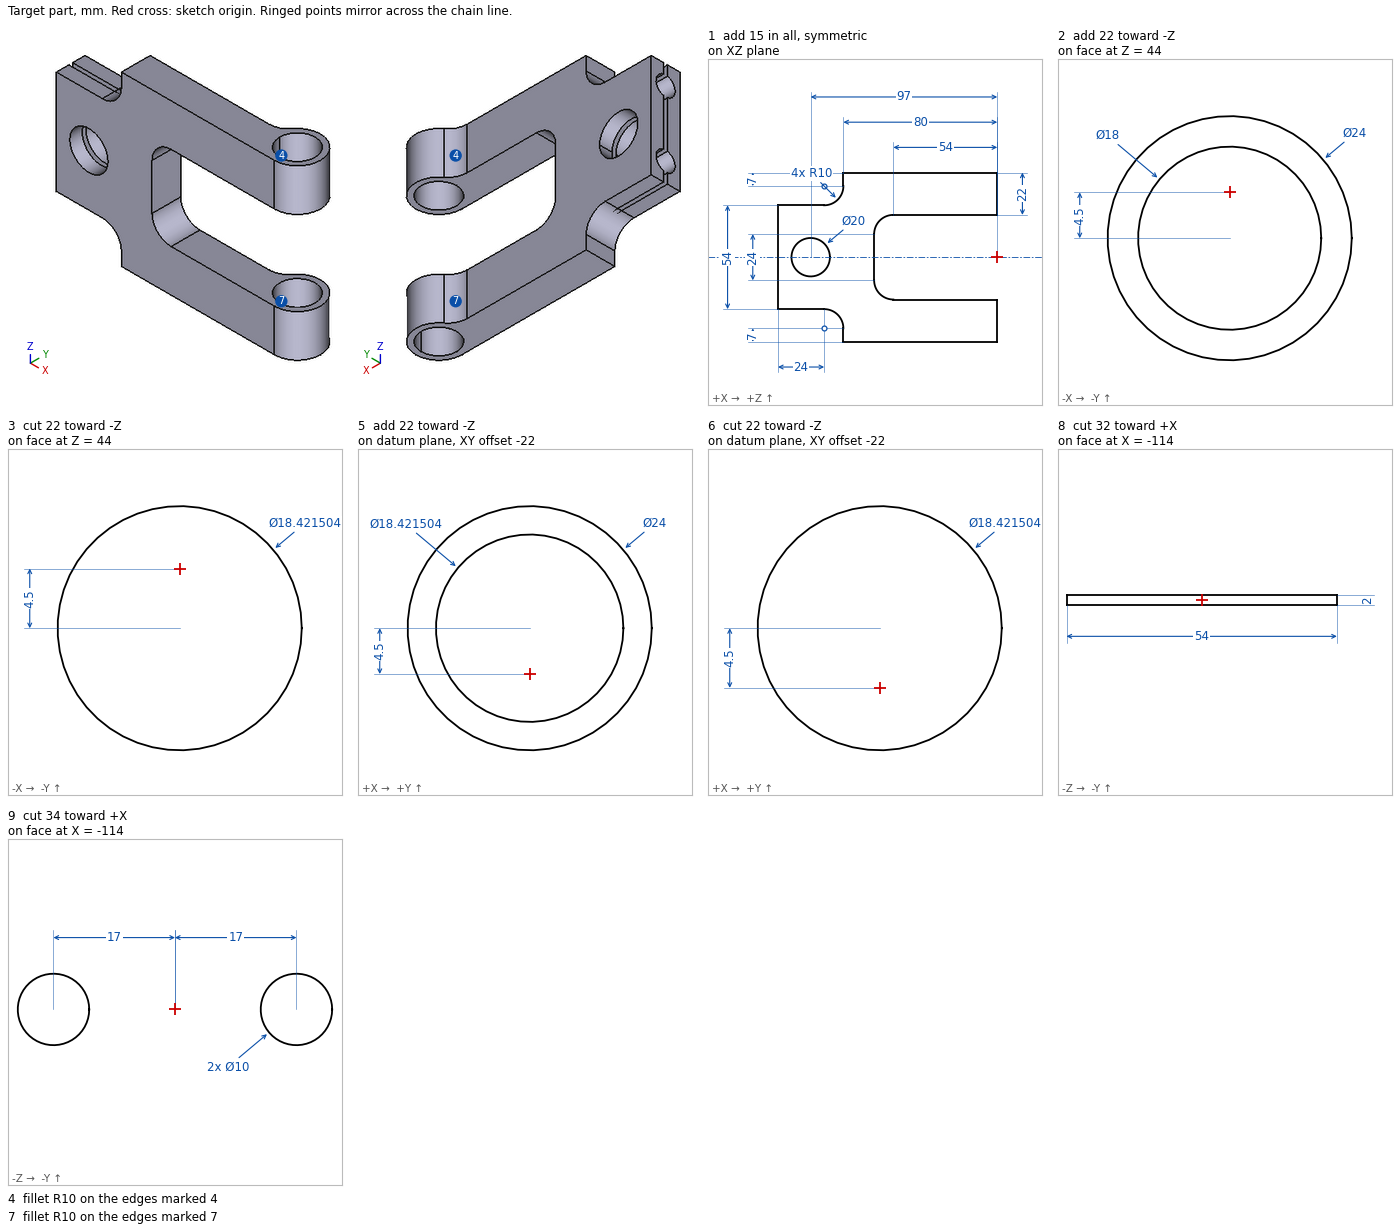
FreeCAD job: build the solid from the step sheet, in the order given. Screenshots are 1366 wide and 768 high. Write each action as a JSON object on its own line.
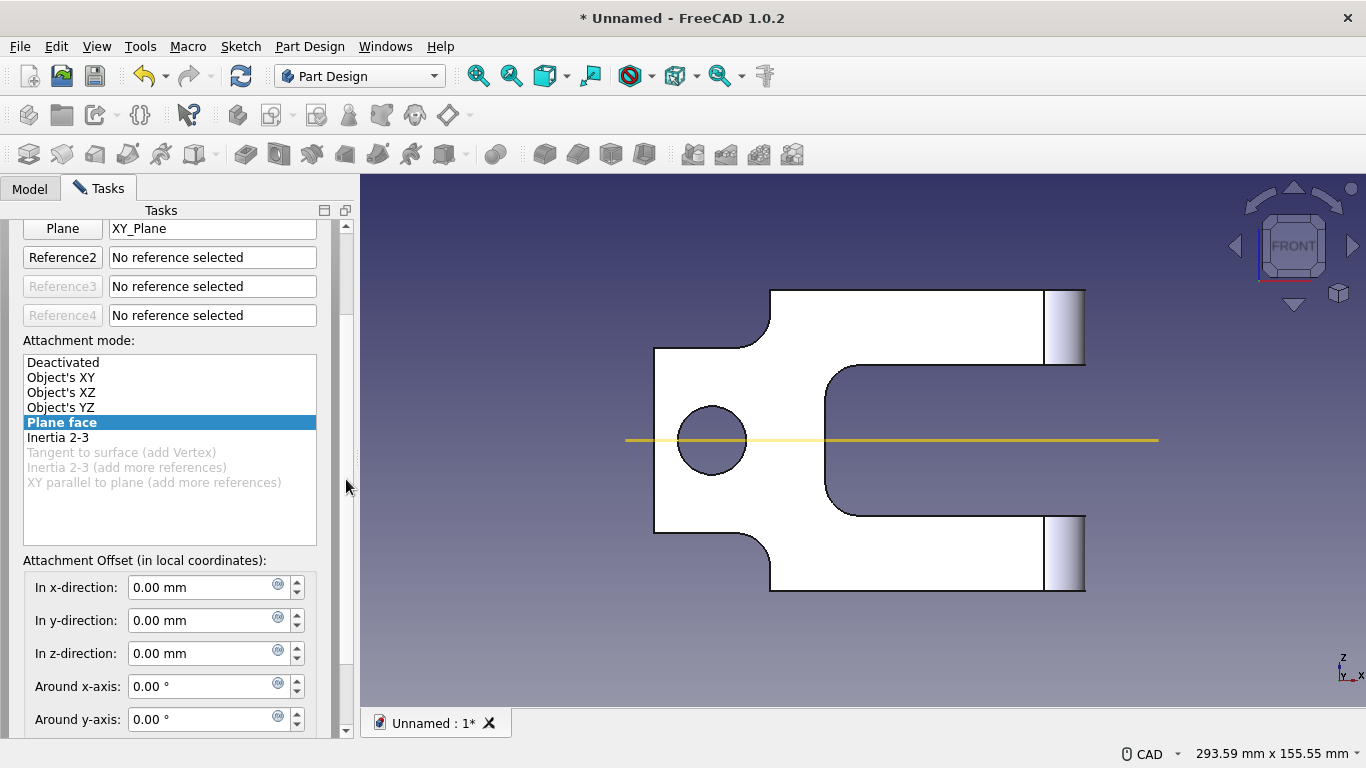
{"action": "triple_click", "coordinate": [210, 654]}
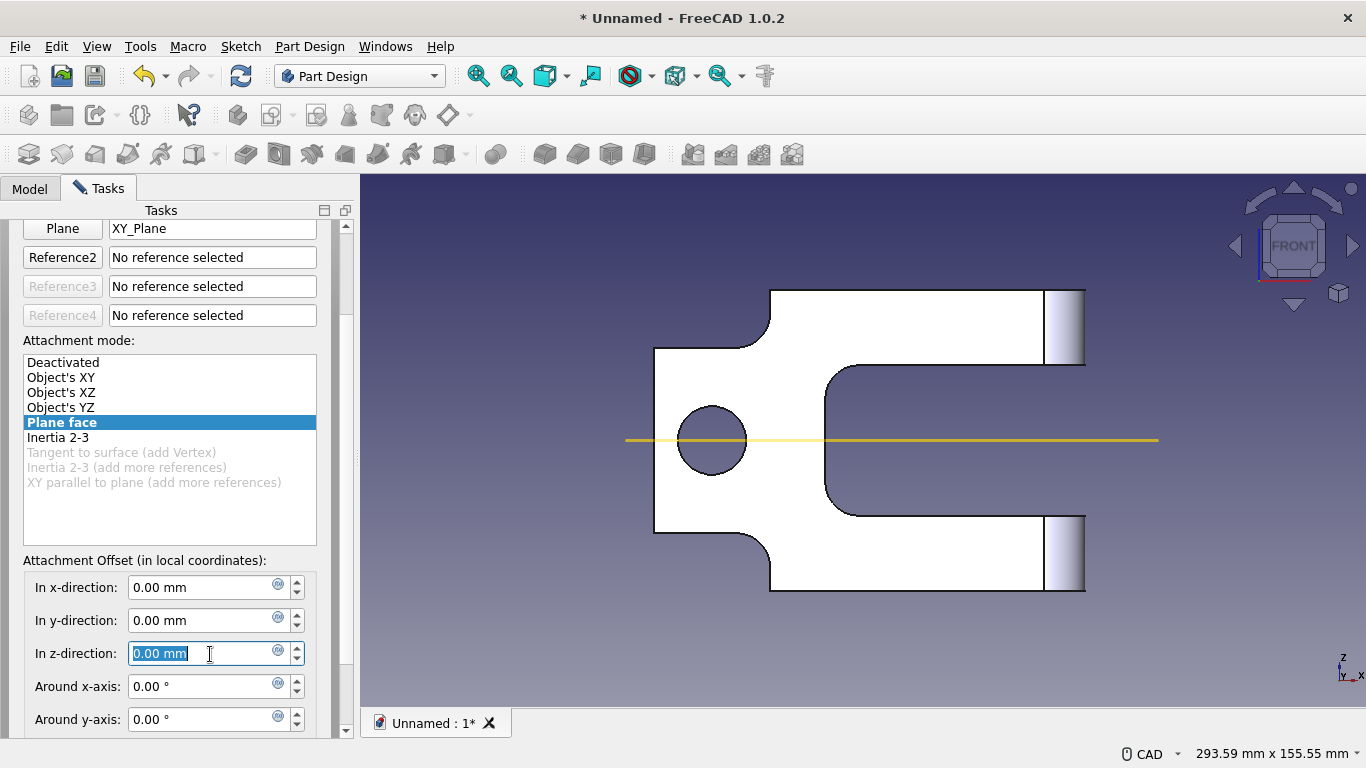
{"action": "type", "text": "-22"}
{"action": "key", "text": "Tab"}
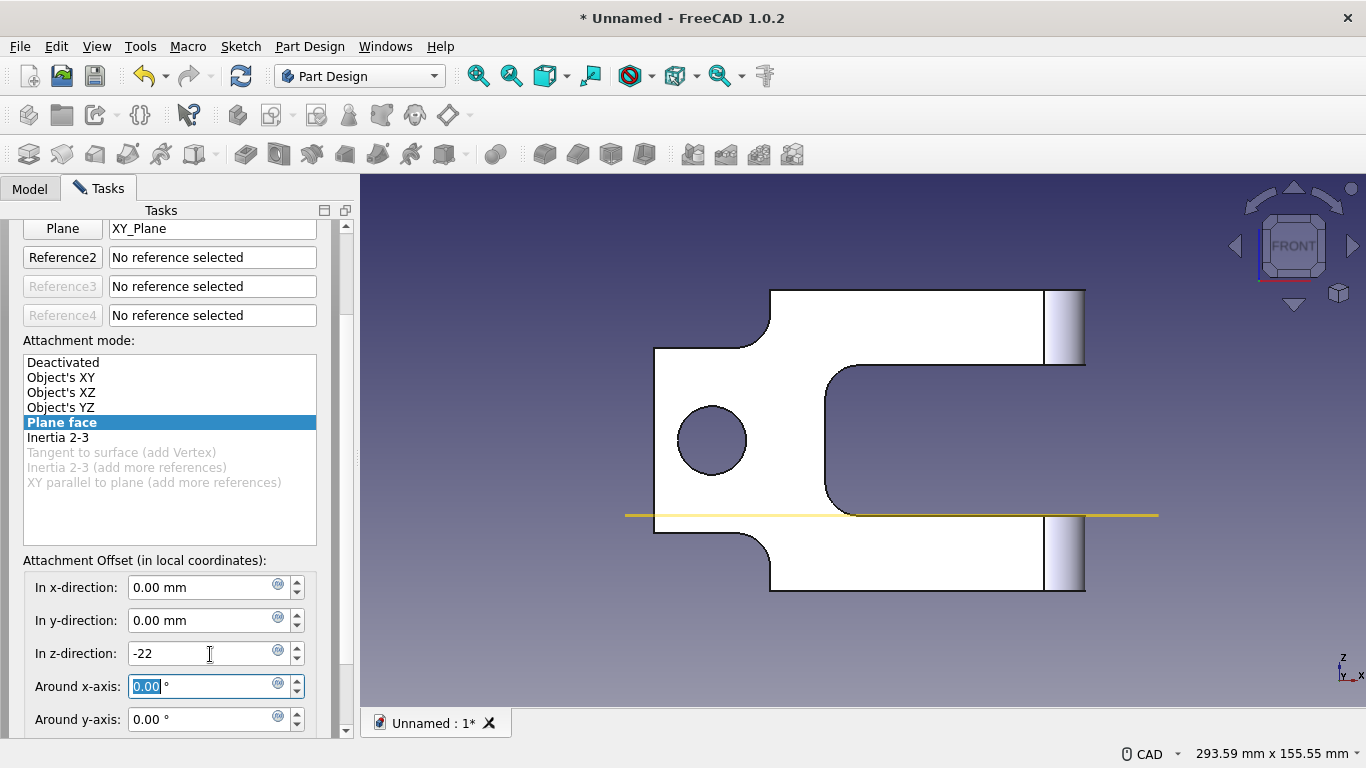
{"action": "scroll", "coordinate": [346, 479], "scroll_direction": "up", "scroll_amount": 3}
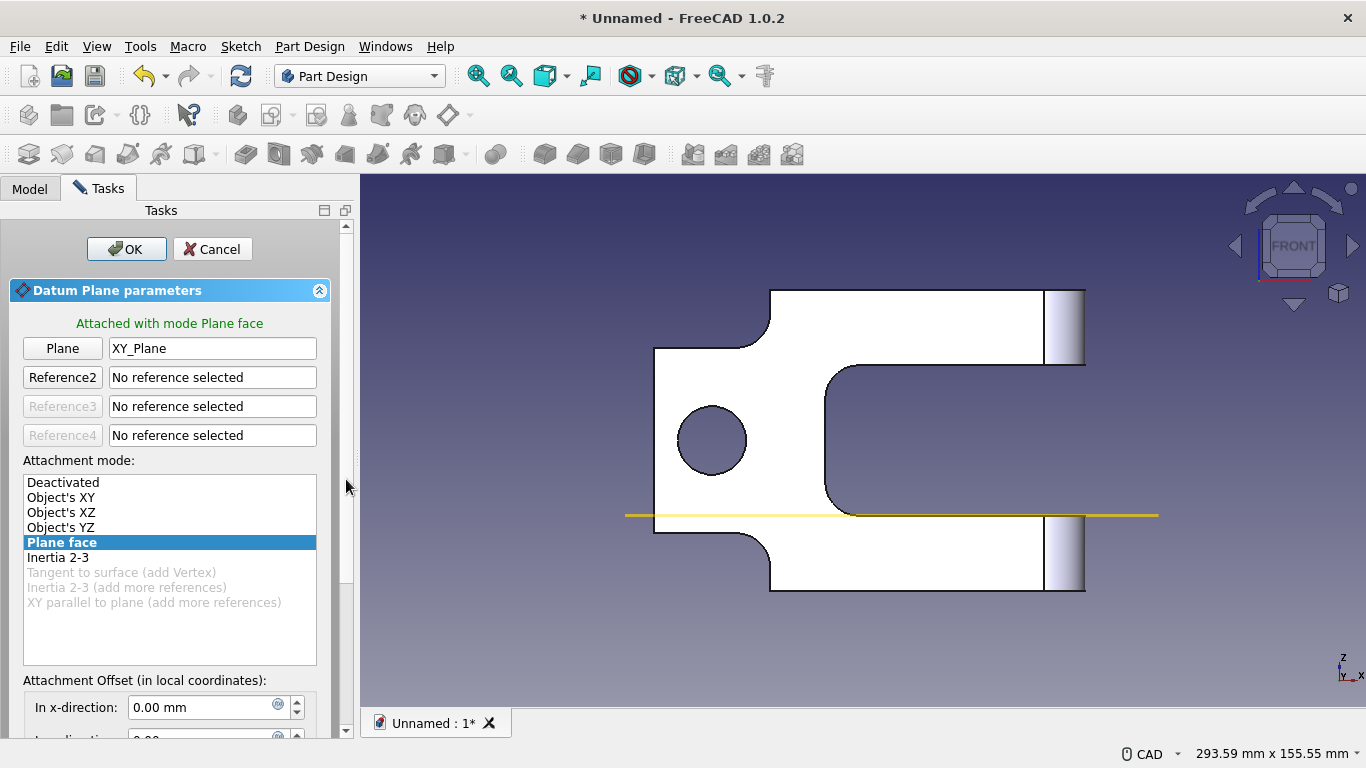
{"action": "left_click", "coordinate": [127, 249]}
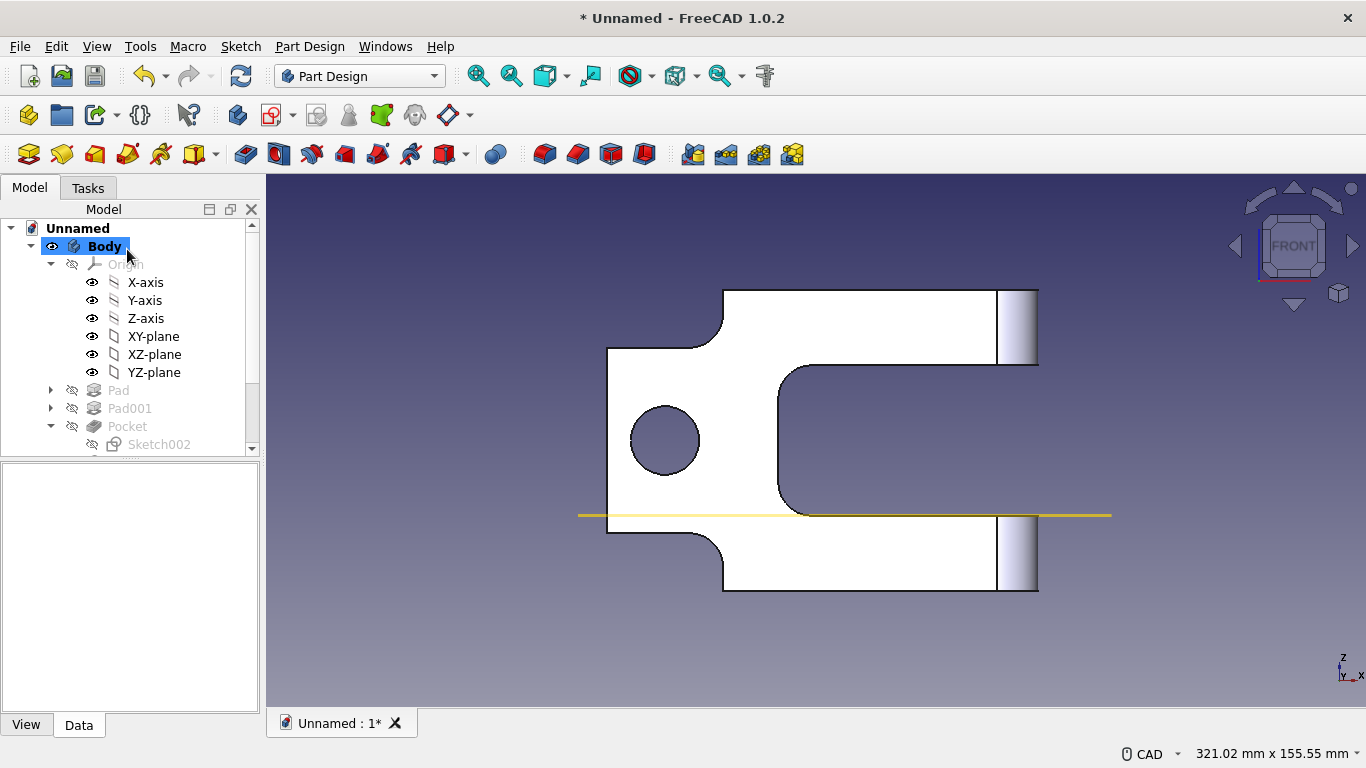
{"action": "scroll", "coordinate": [101, 332], "scroll_direction": "down", "scroll_amount": 3}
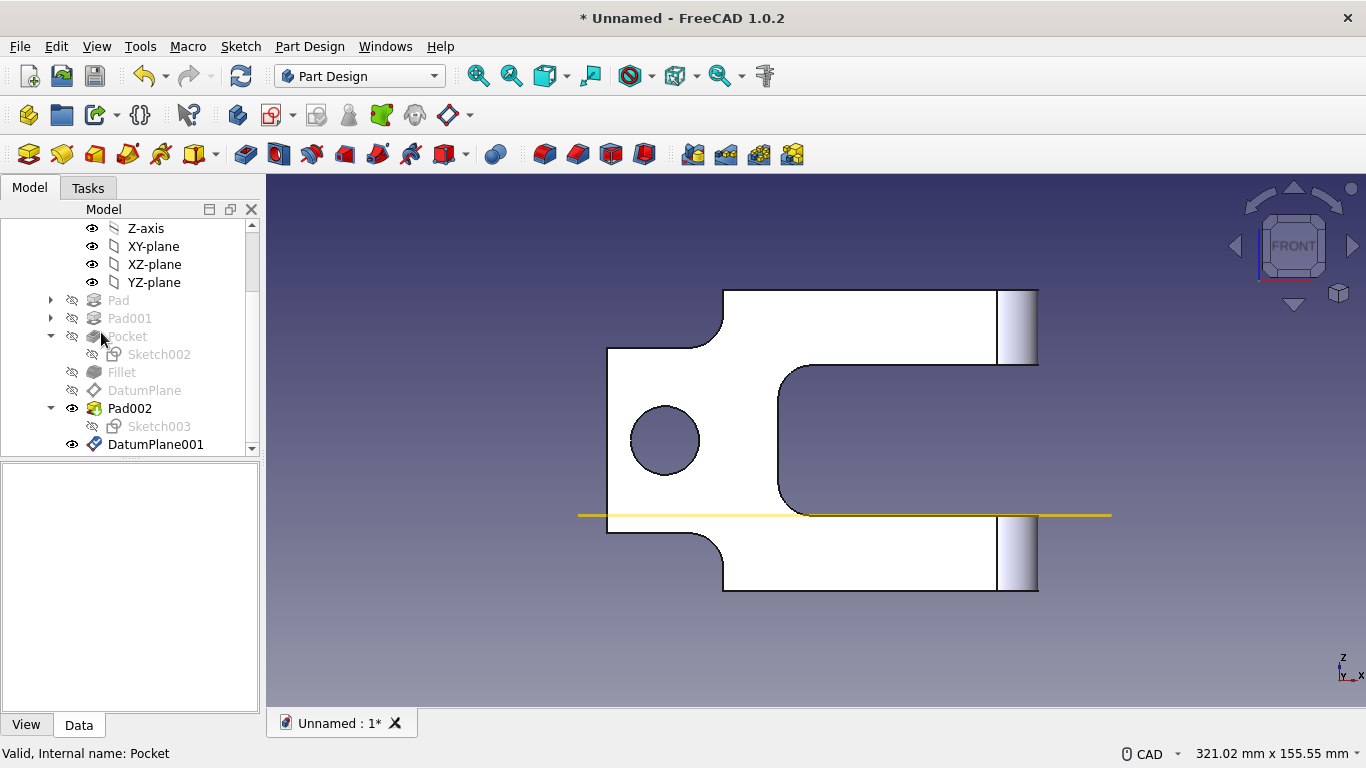
{"action": "left_click", "coordinate": [117, 444]}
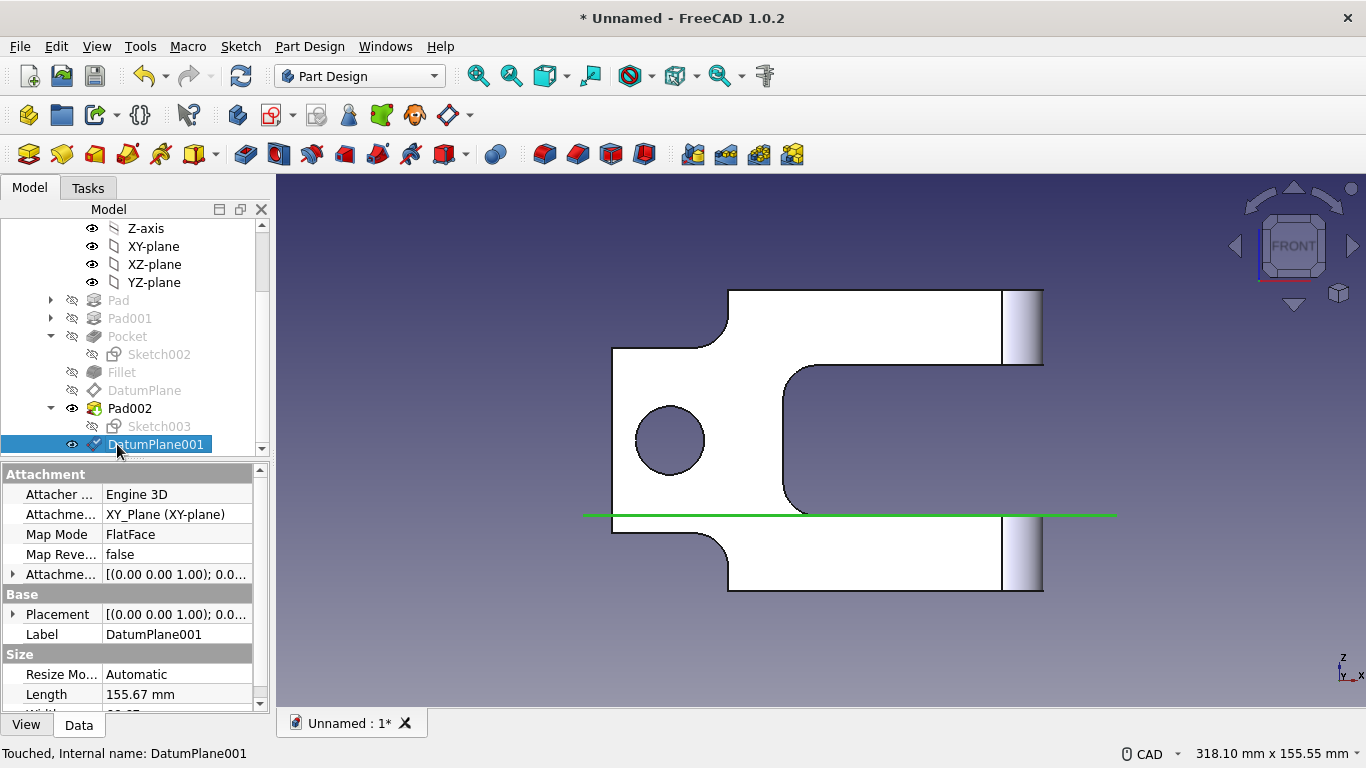
{"action": "left_click", "coordinate": [270, 116]}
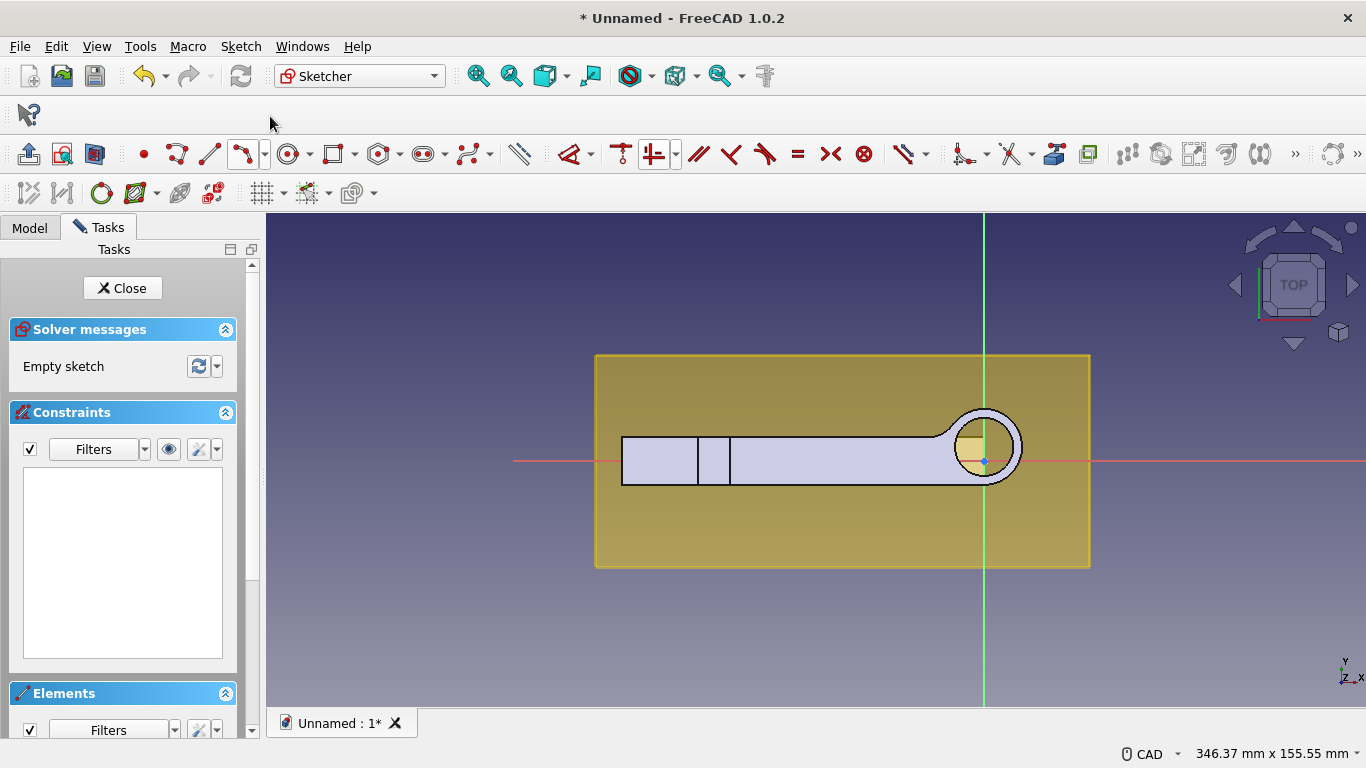
{"action": "left_click", "coordinate": [95, 154]}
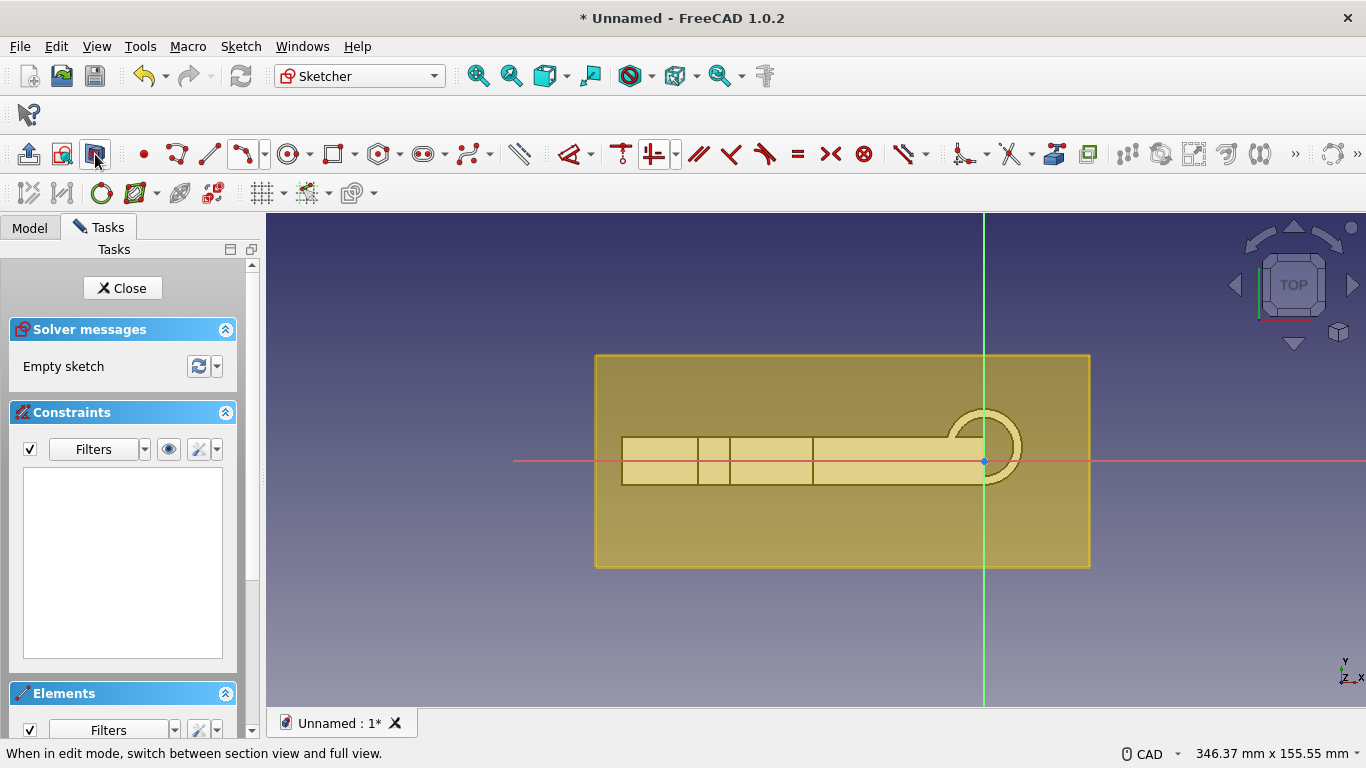
{"action": "scroll", "coordinate": [1044, 444], "scroll_direction": "up", "scroll_amount": 8}